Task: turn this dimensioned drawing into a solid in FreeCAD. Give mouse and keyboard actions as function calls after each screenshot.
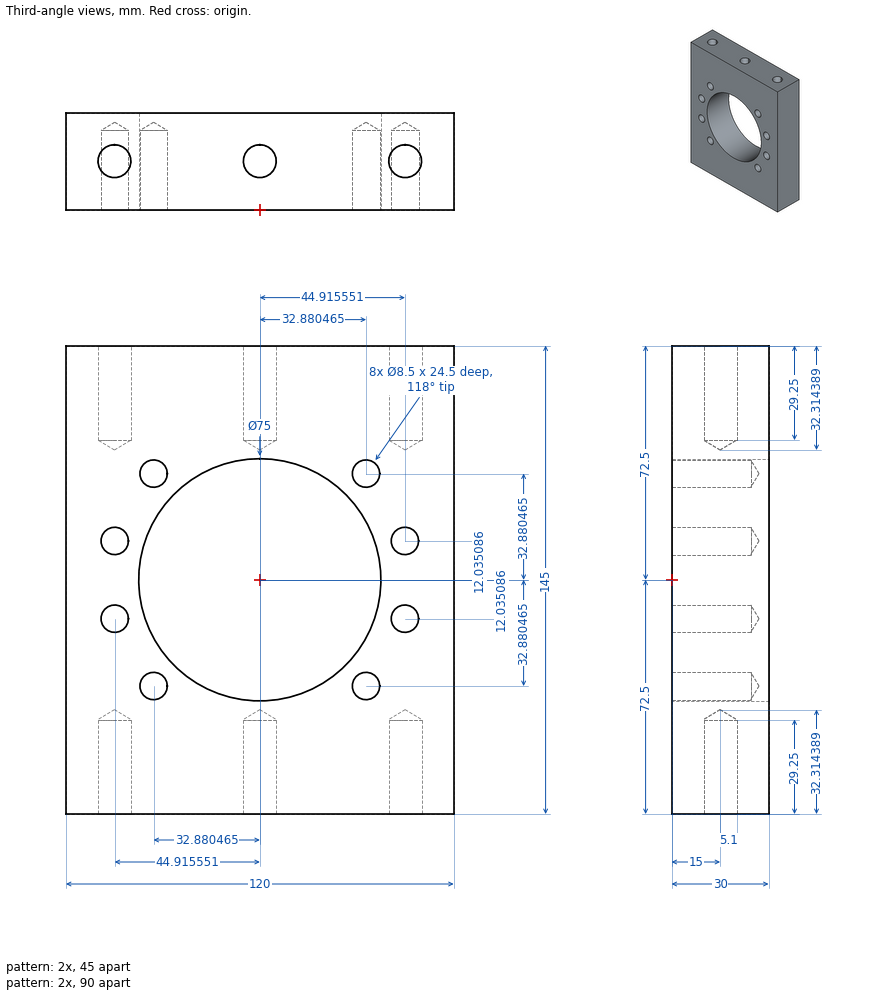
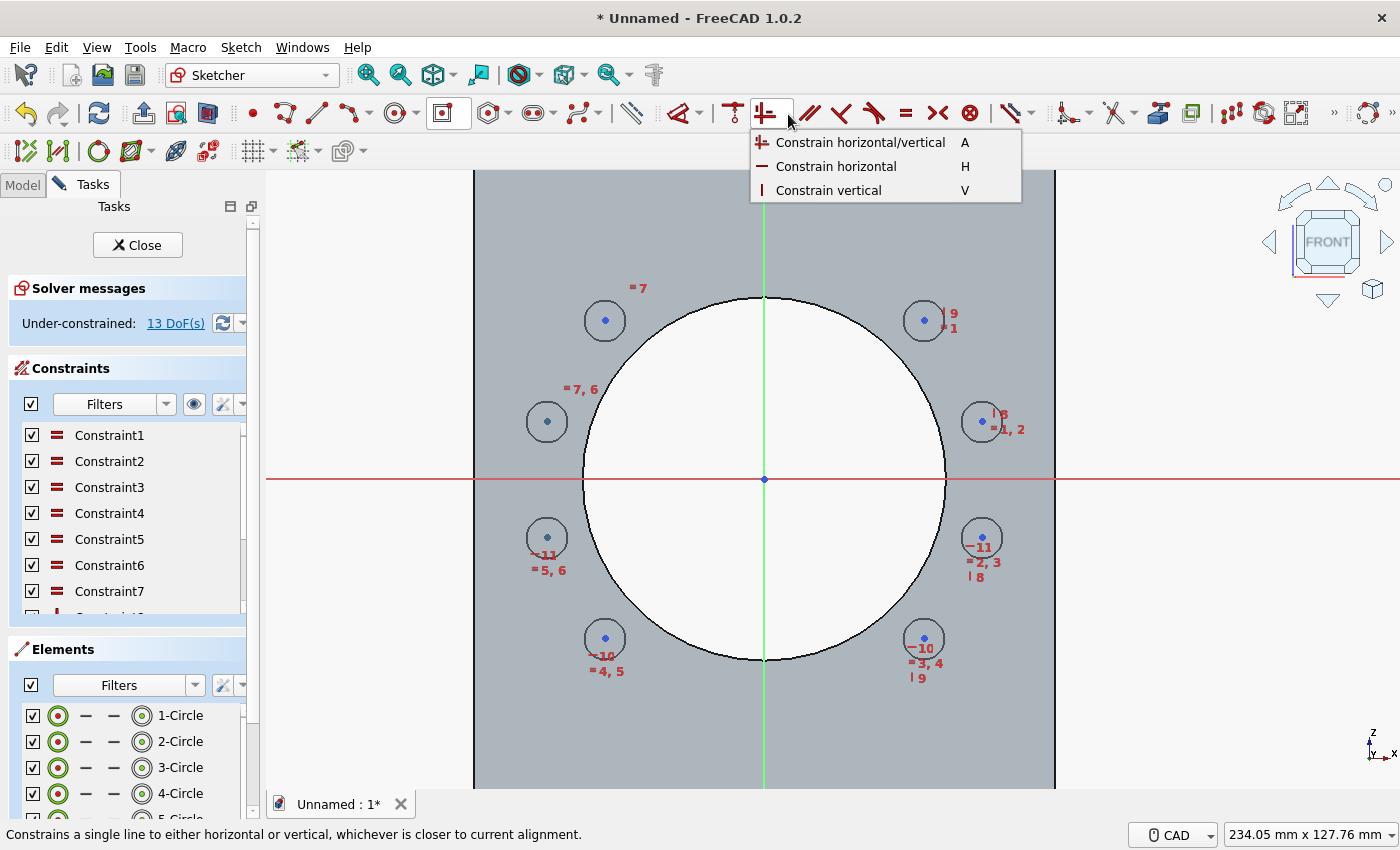
click(886, 190)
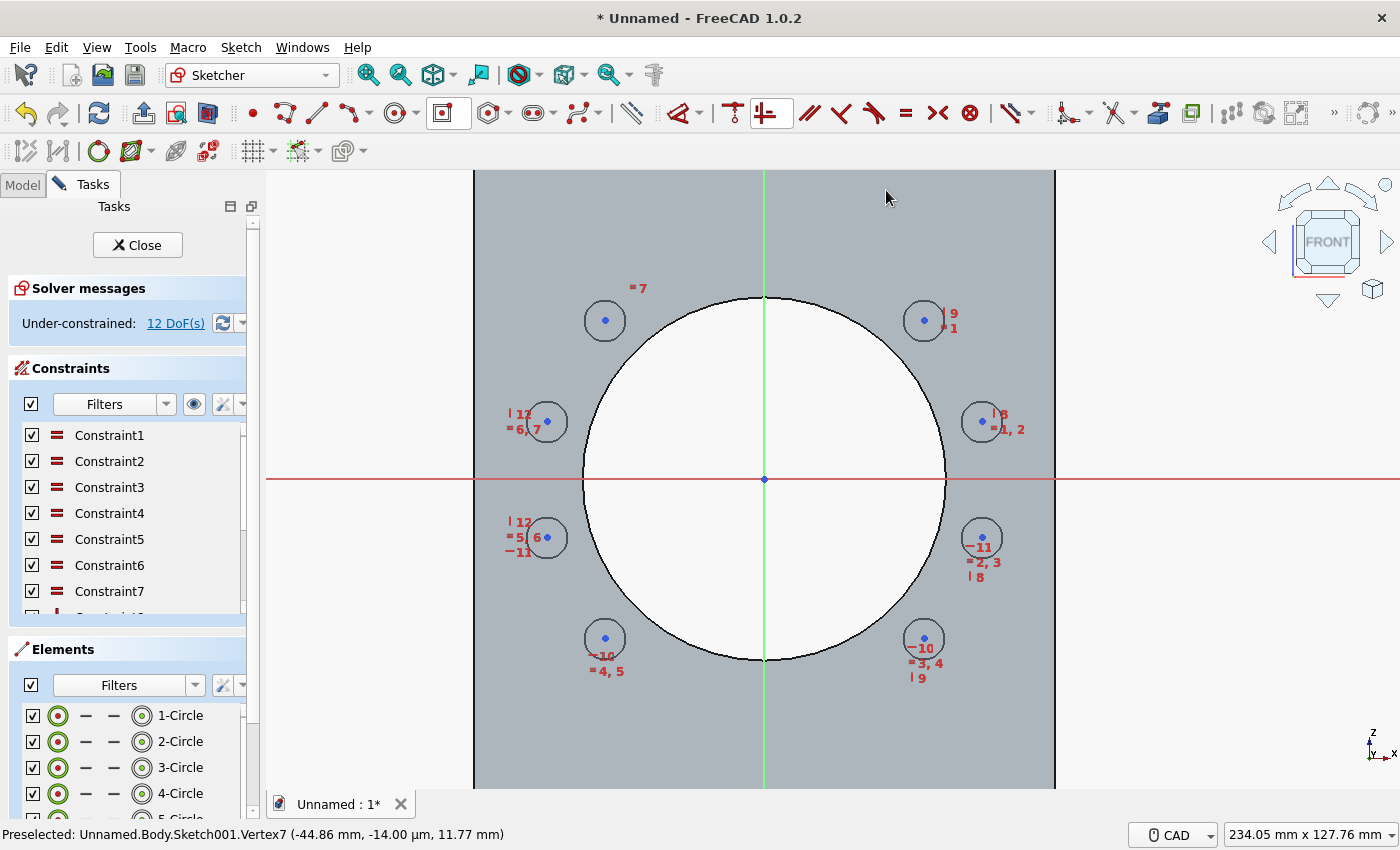
click(982, 422)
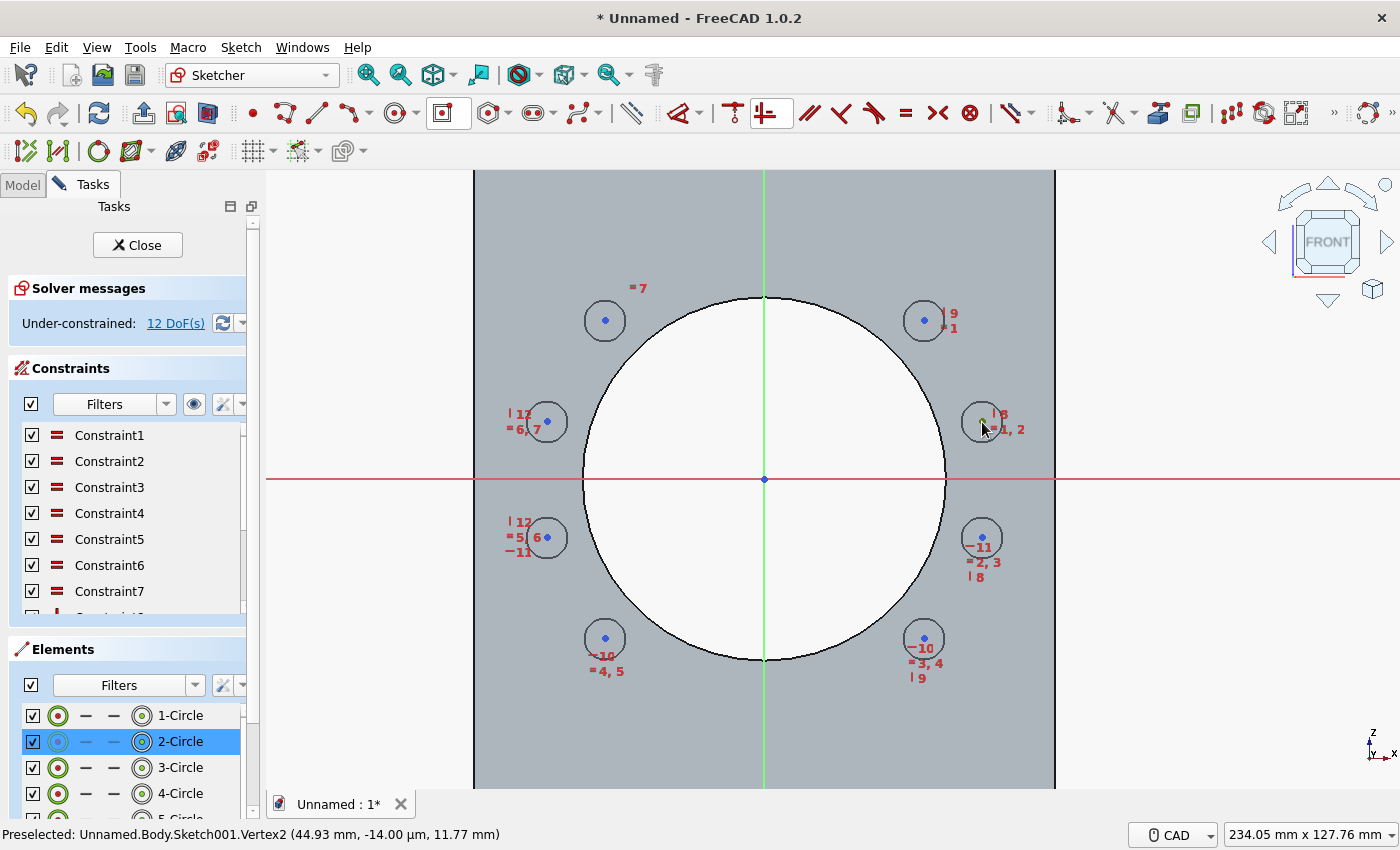
click(547, 422)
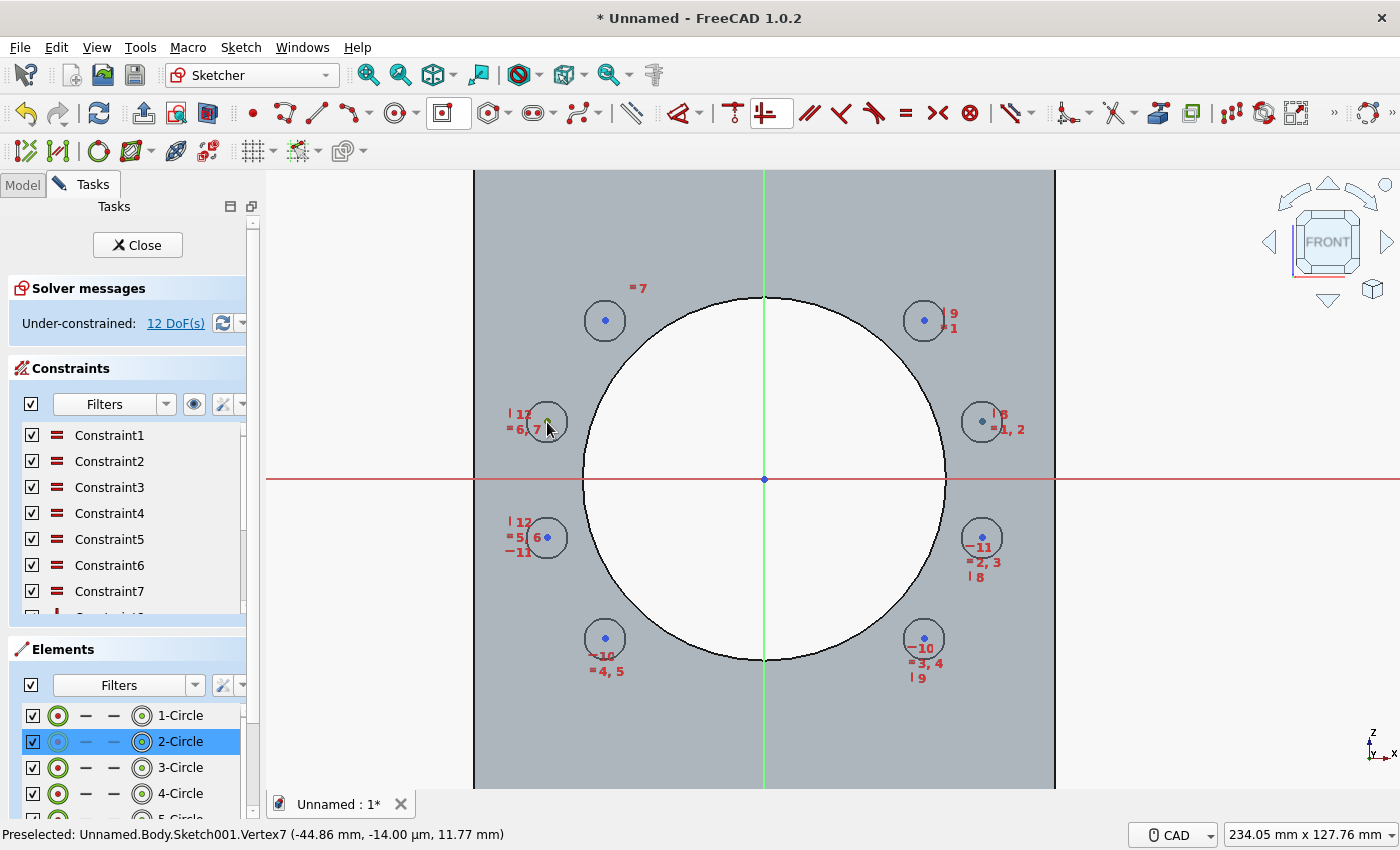
key(h)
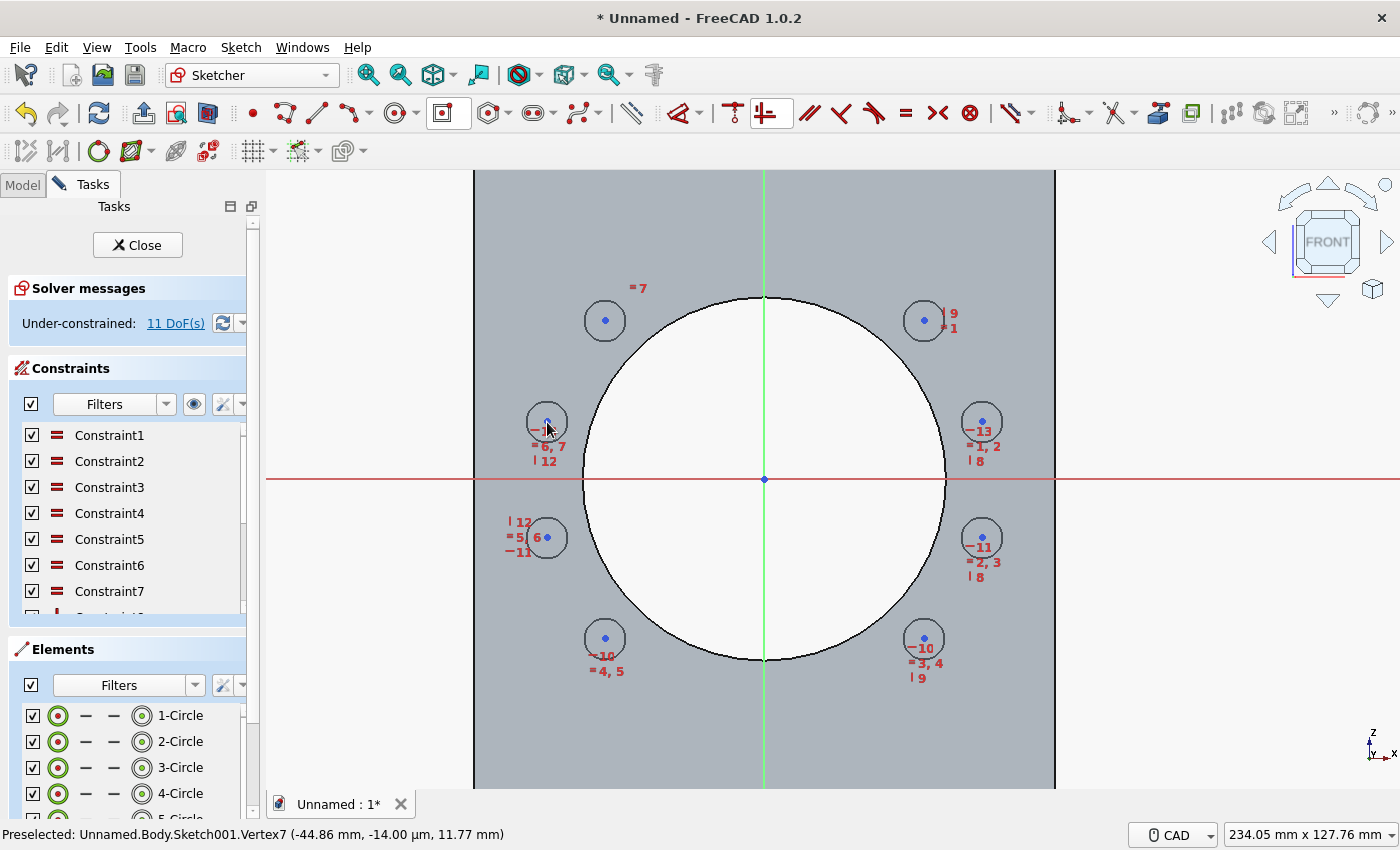
click(605, 639)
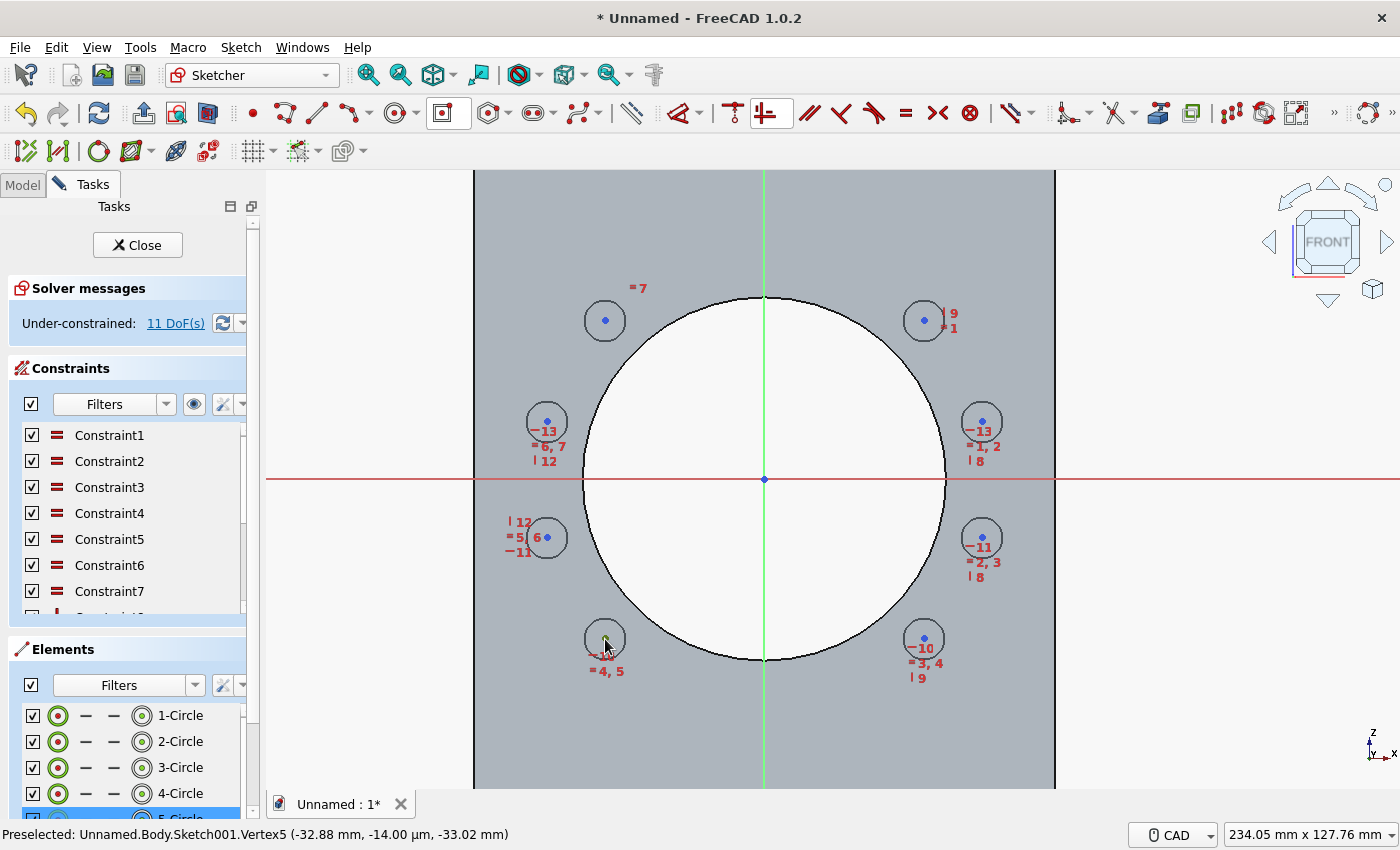
click(605, 321)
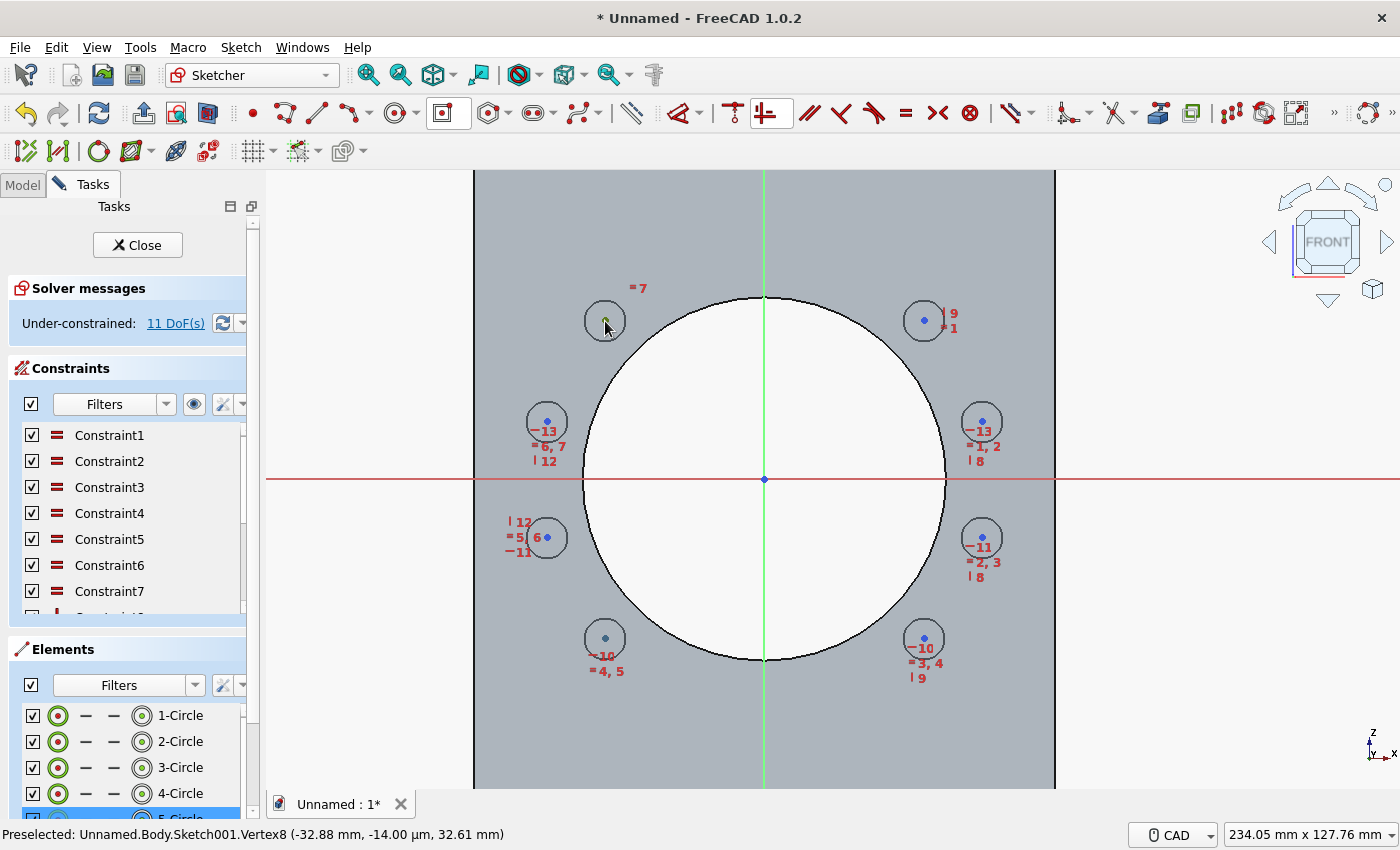
click(788, 114)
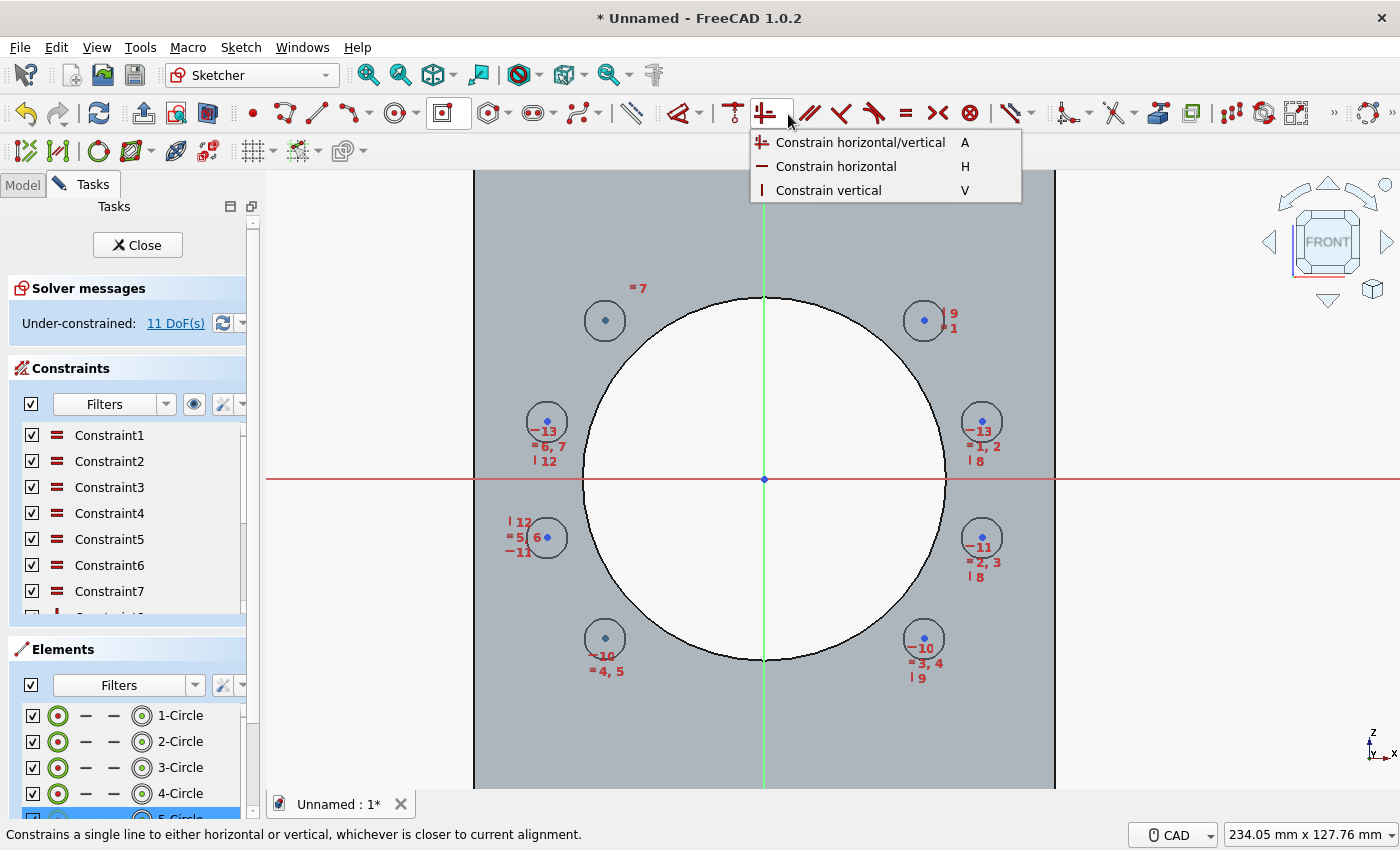
click(886, 190)